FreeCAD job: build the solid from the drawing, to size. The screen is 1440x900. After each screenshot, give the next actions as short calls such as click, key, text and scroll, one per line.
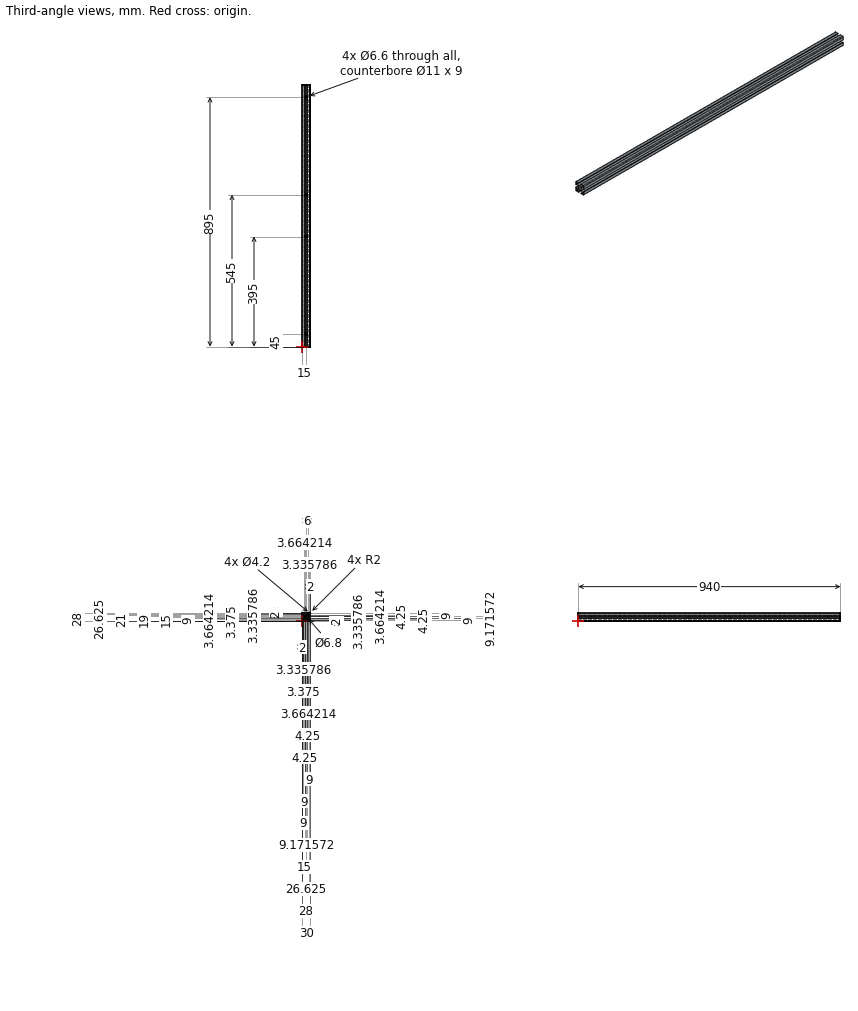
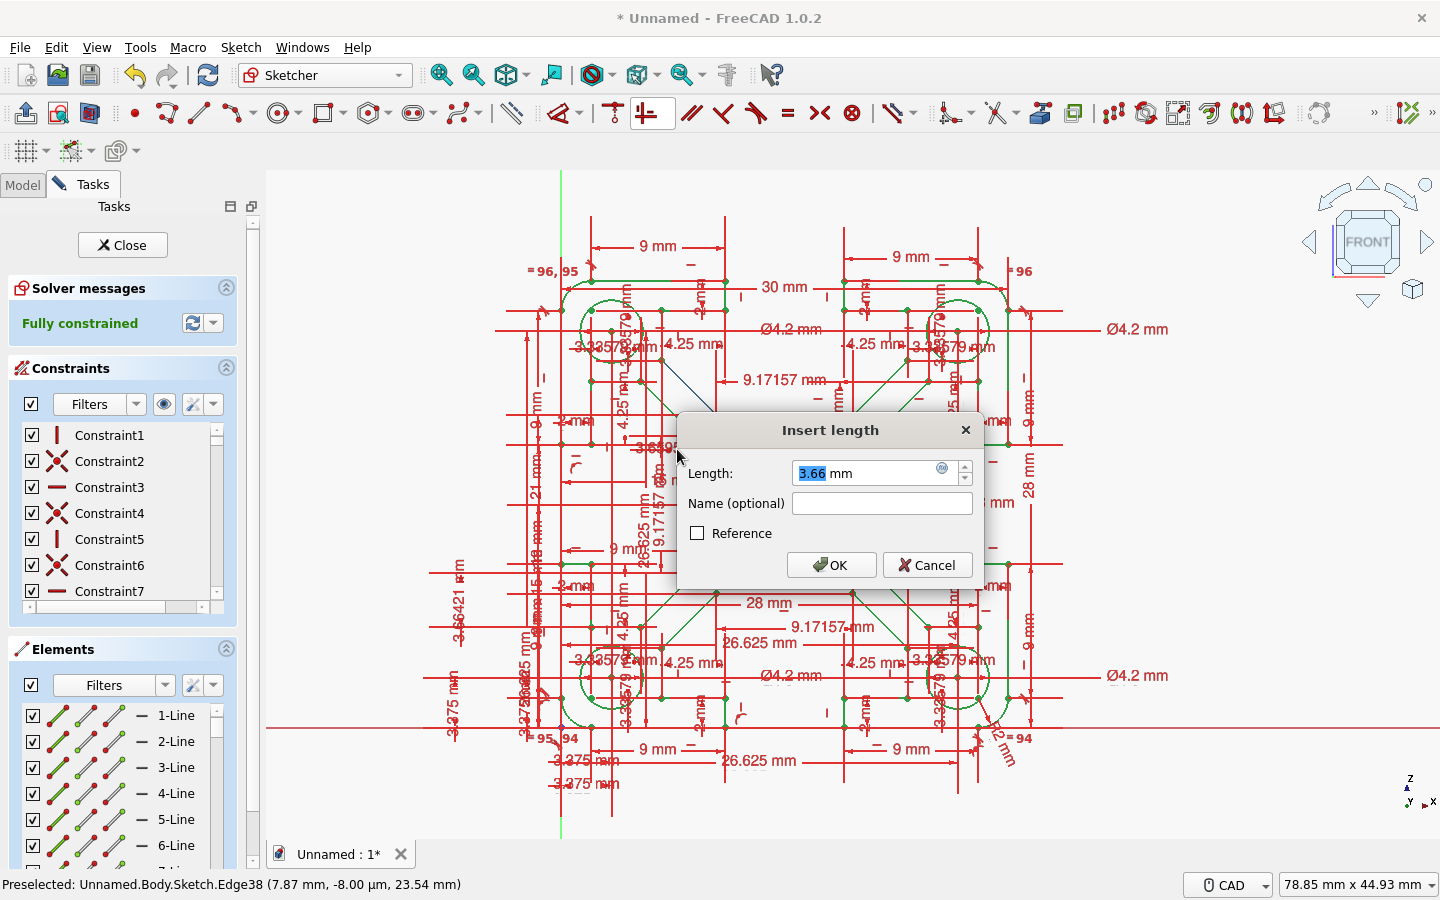
text(3.664214)
key(Return)
key(Escape)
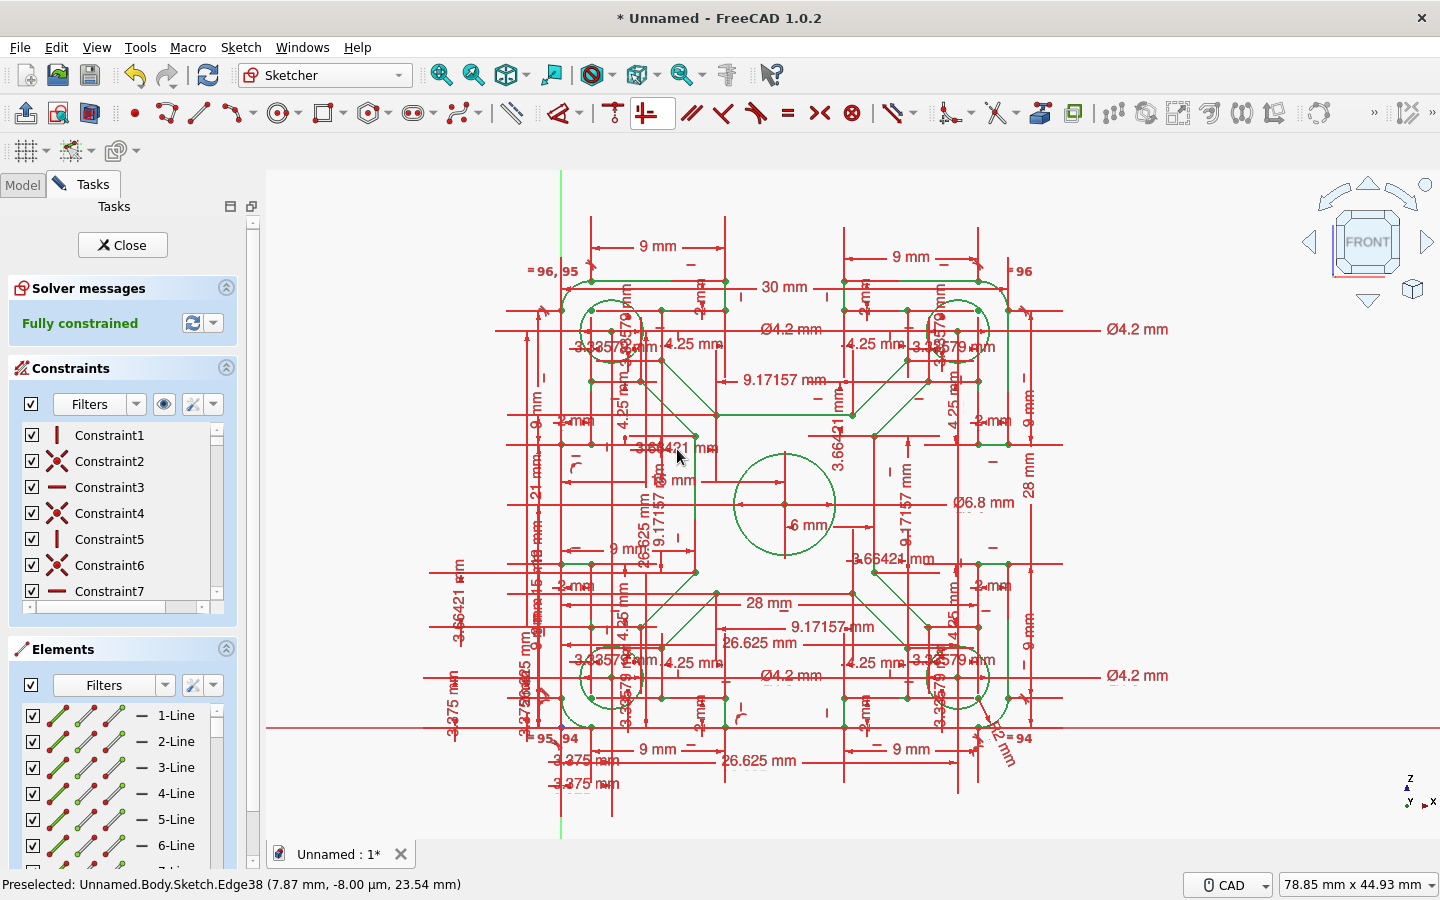
click(123, 245)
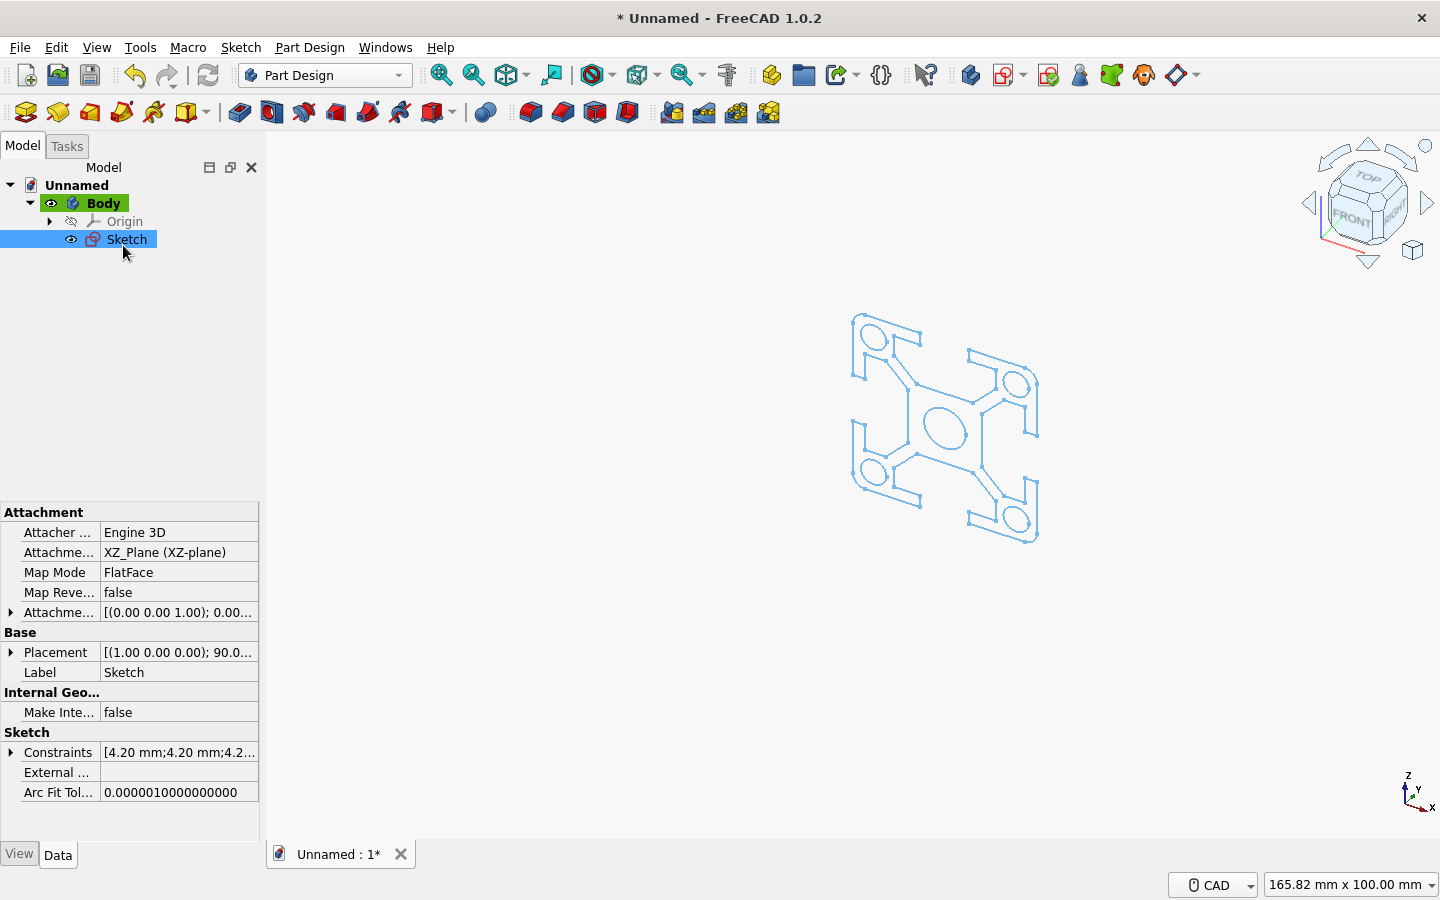
click(26, 112)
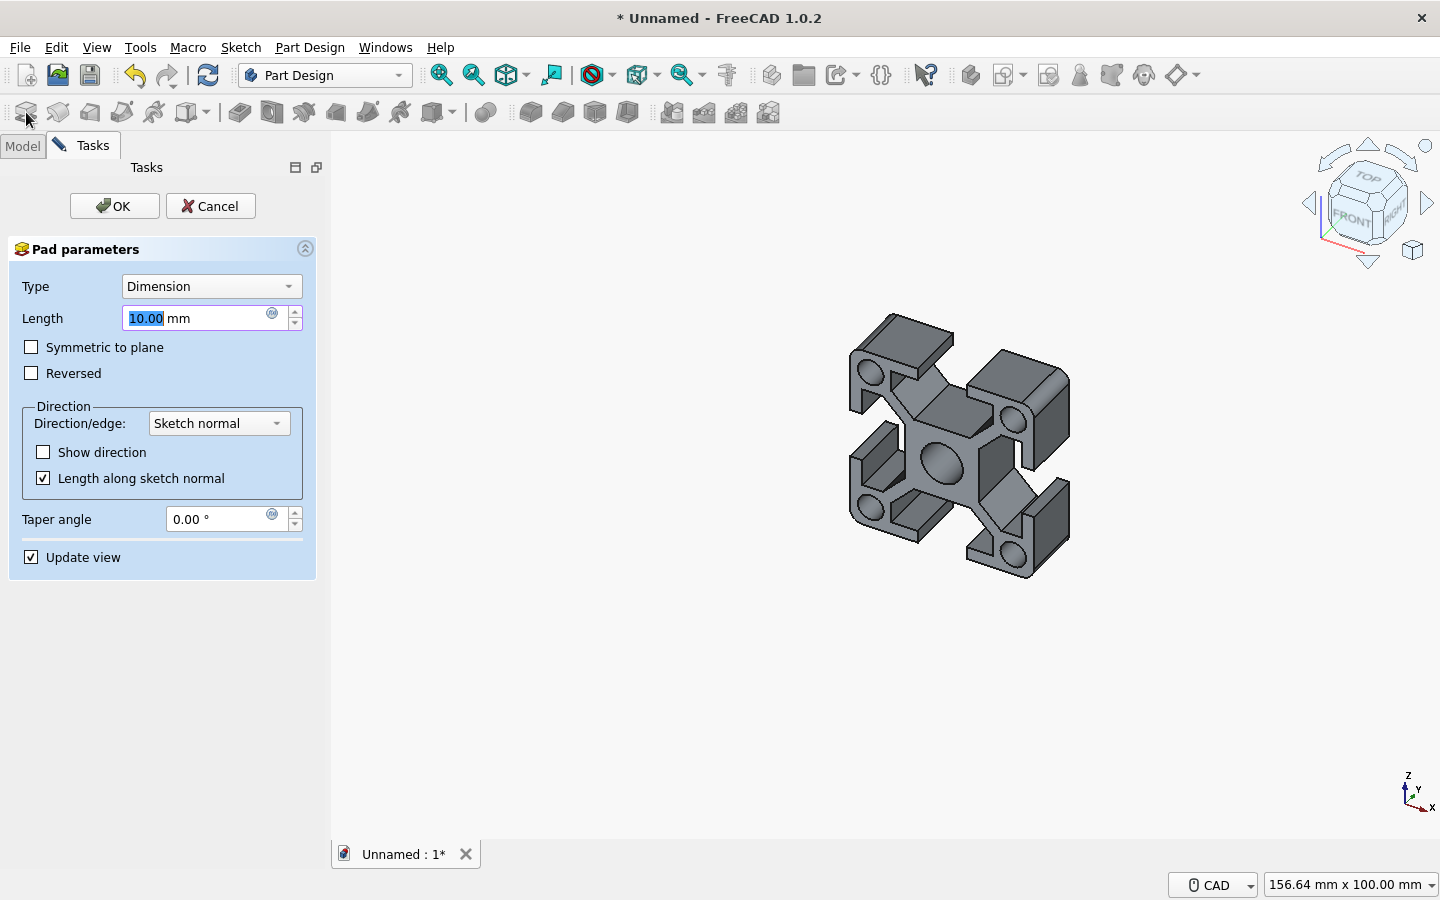
text(940)
key(Tab)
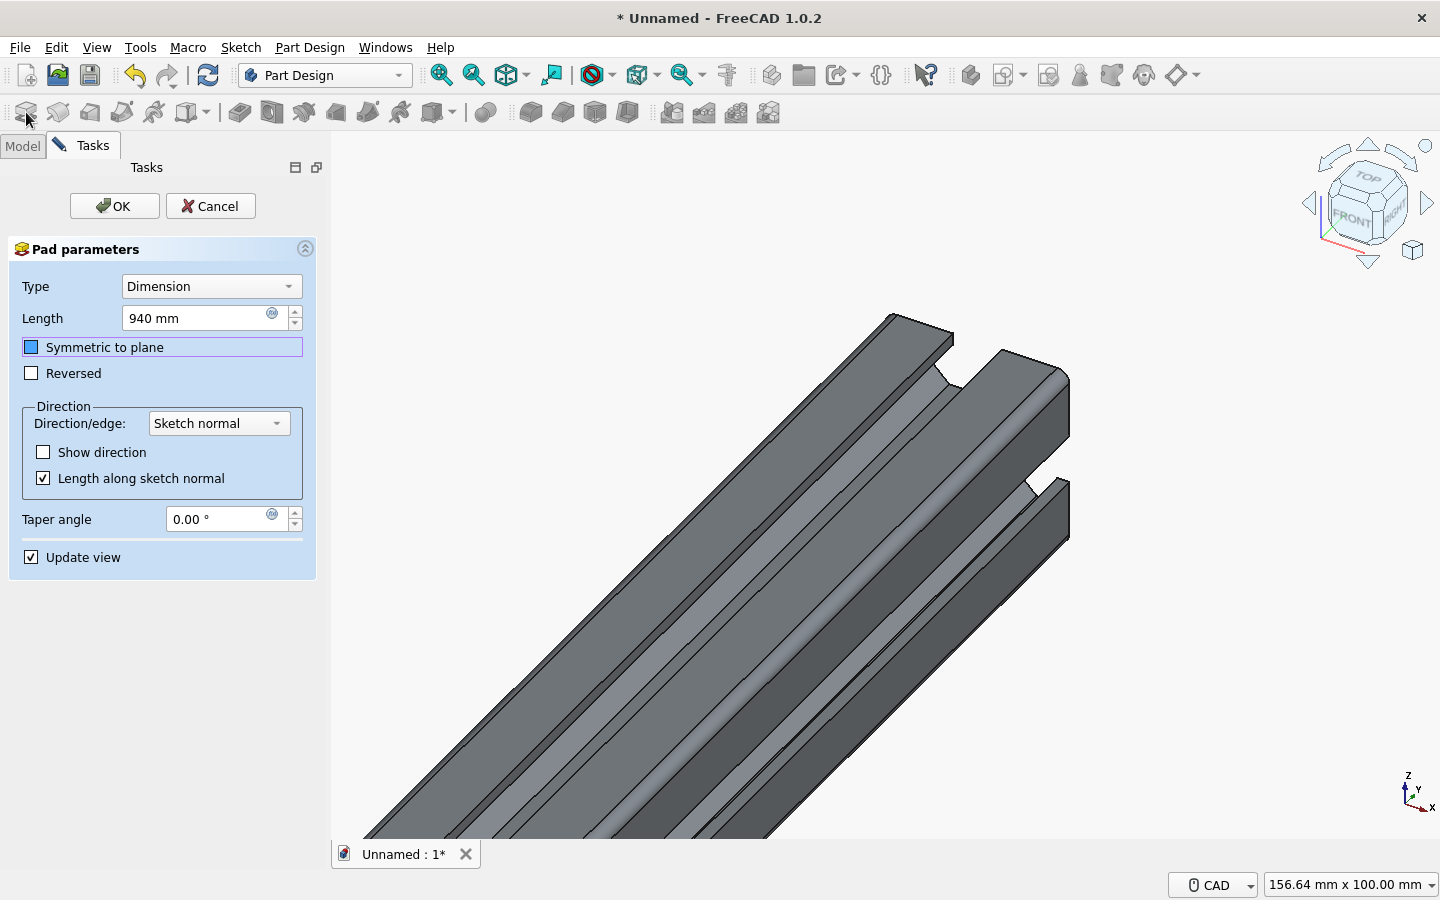
click(30, 373)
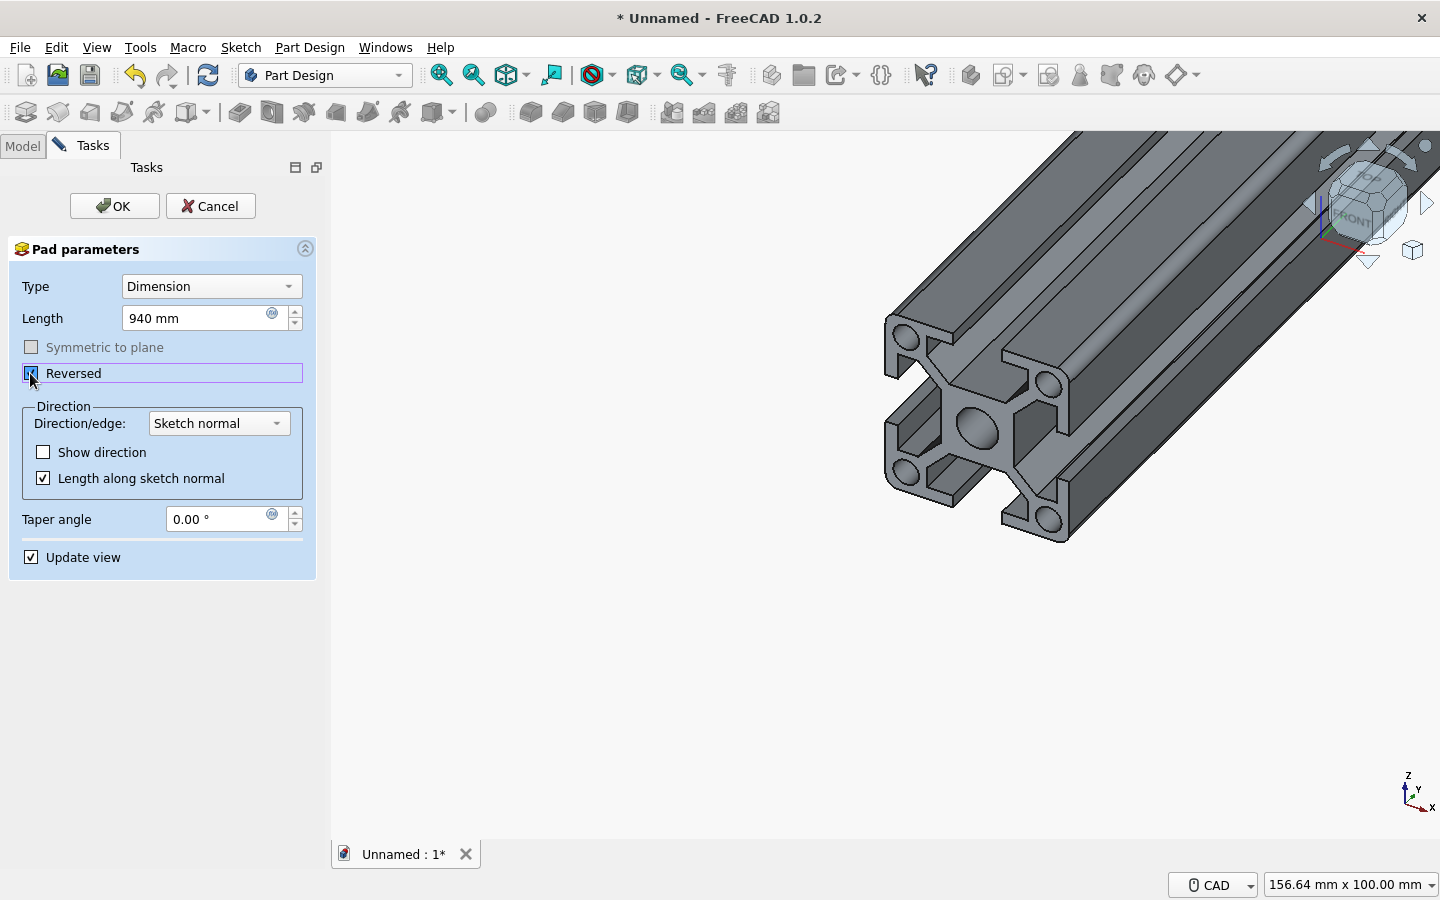
click(115, 206)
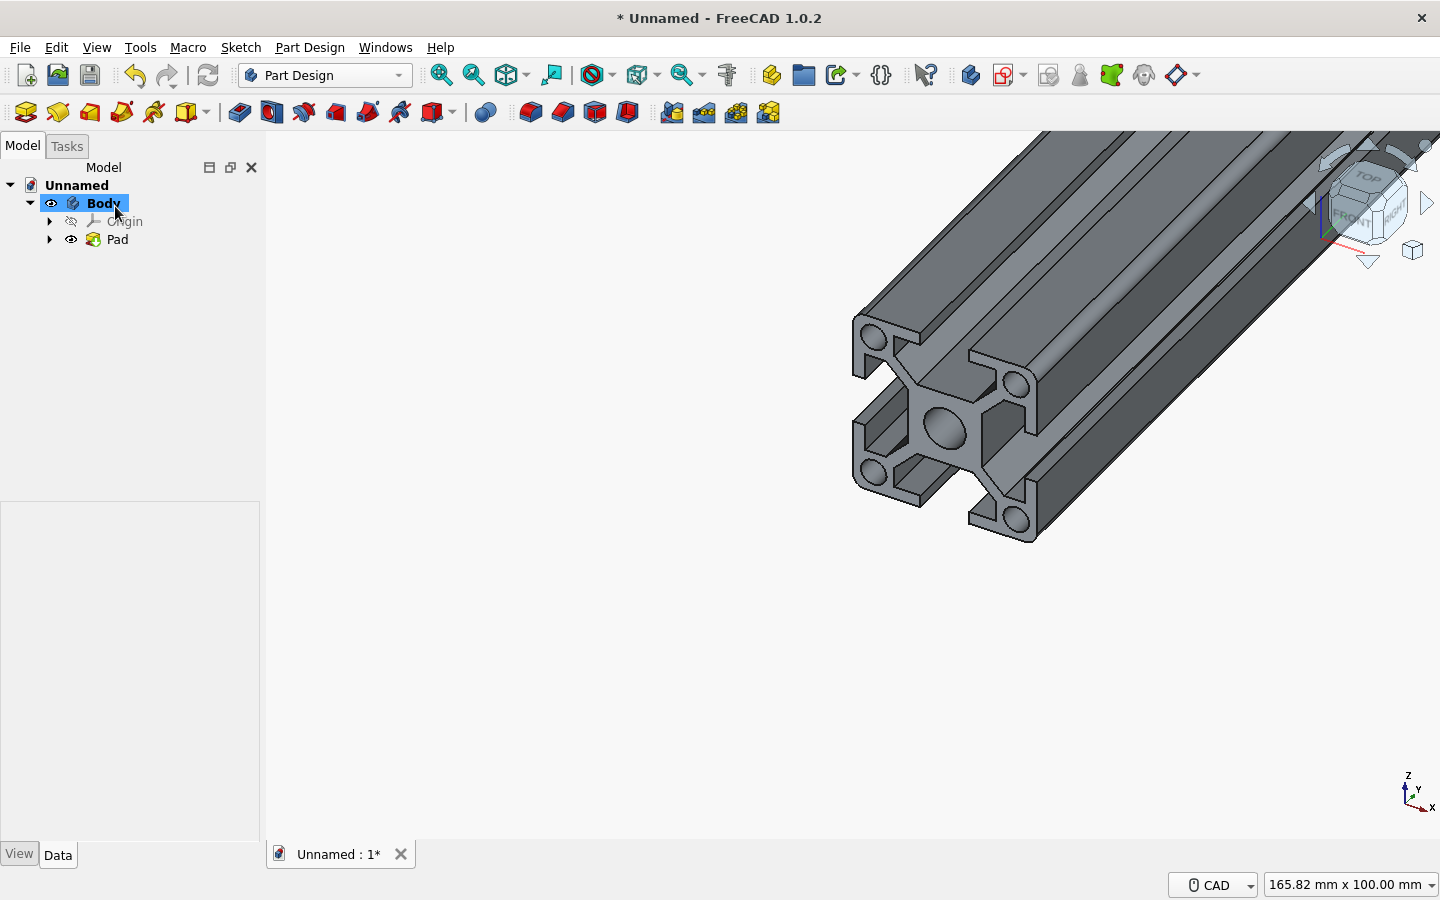
click(442, 76)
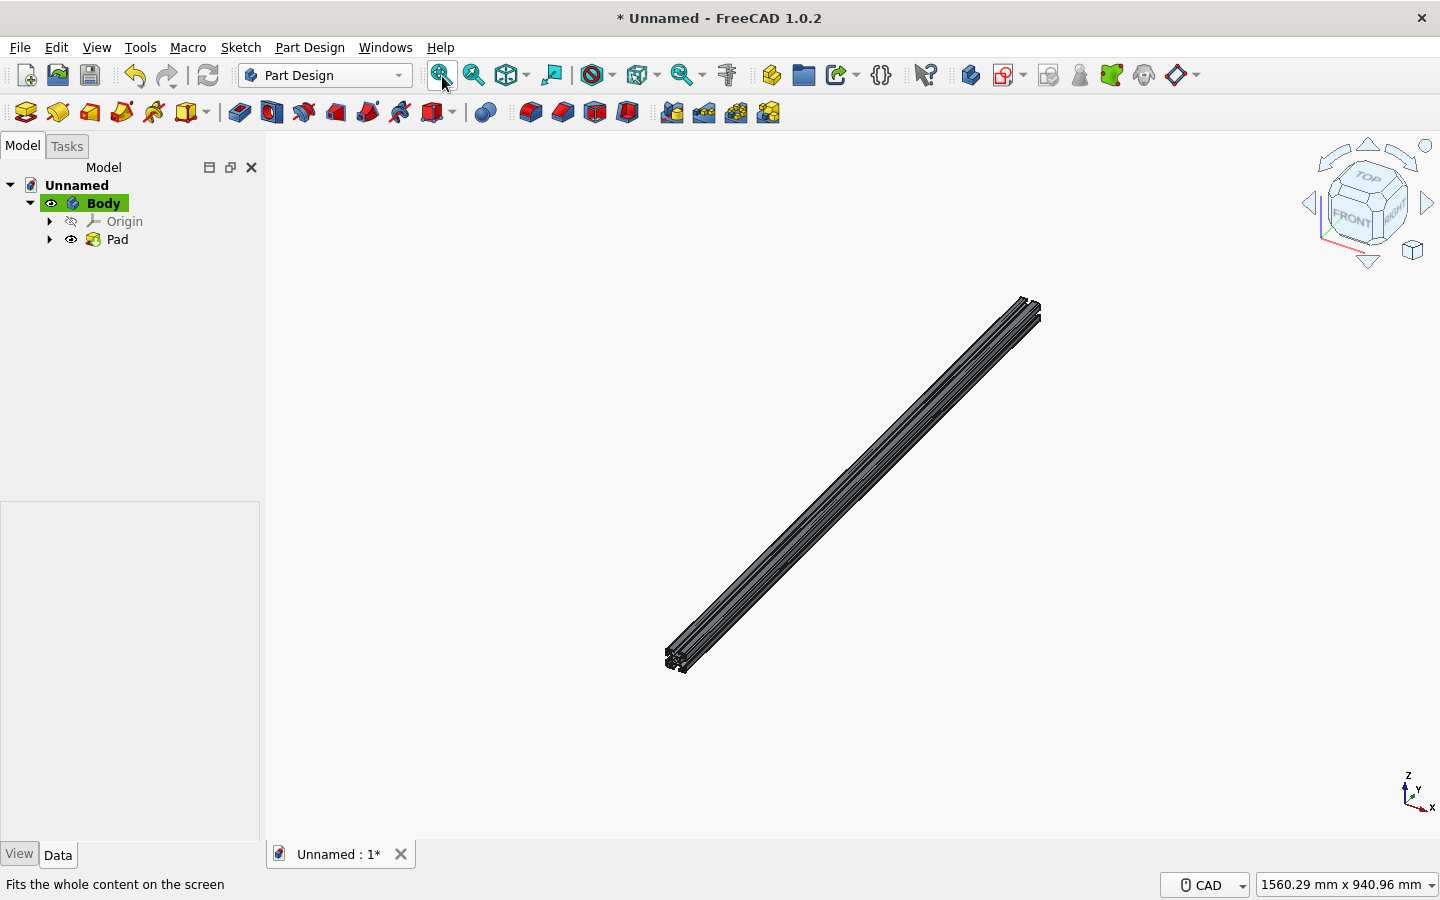
click(1004, 76)